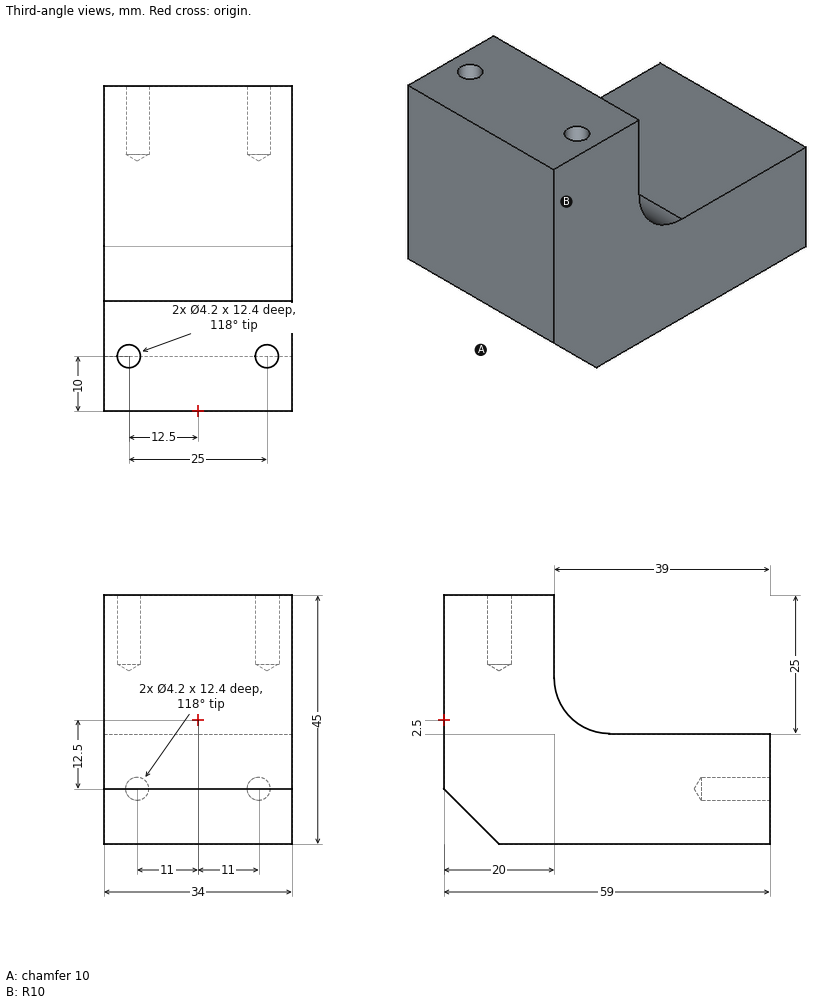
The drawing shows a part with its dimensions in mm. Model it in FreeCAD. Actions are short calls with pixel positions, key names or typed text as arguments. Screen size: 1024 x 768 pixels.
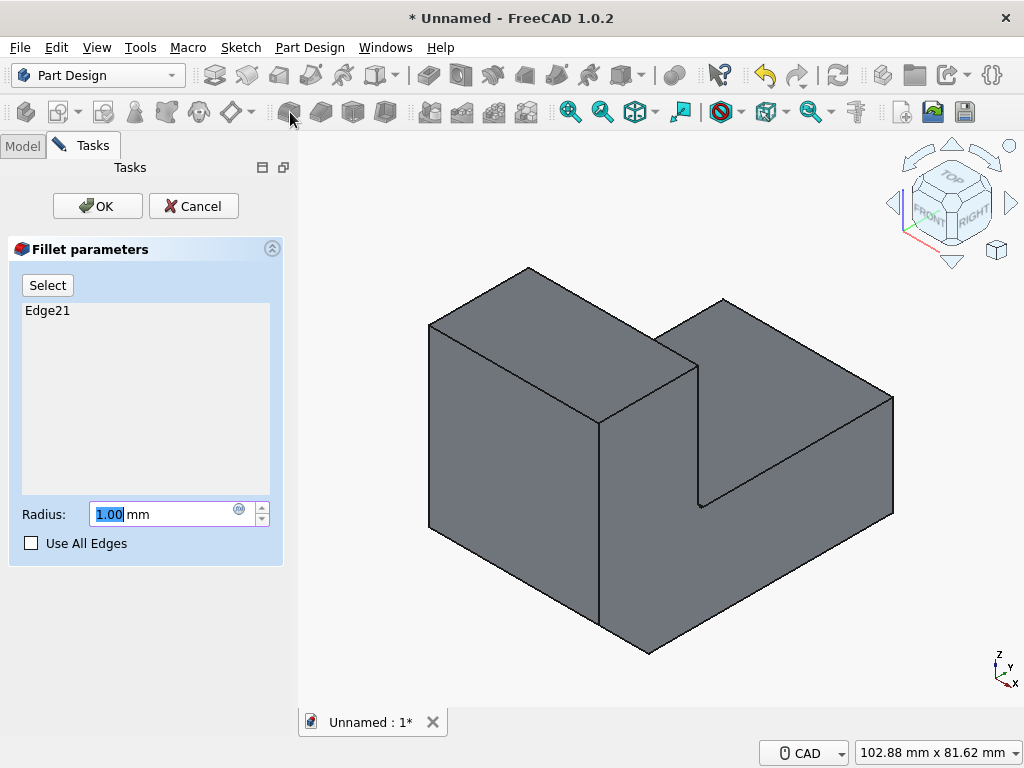
text(10)
key(Tab)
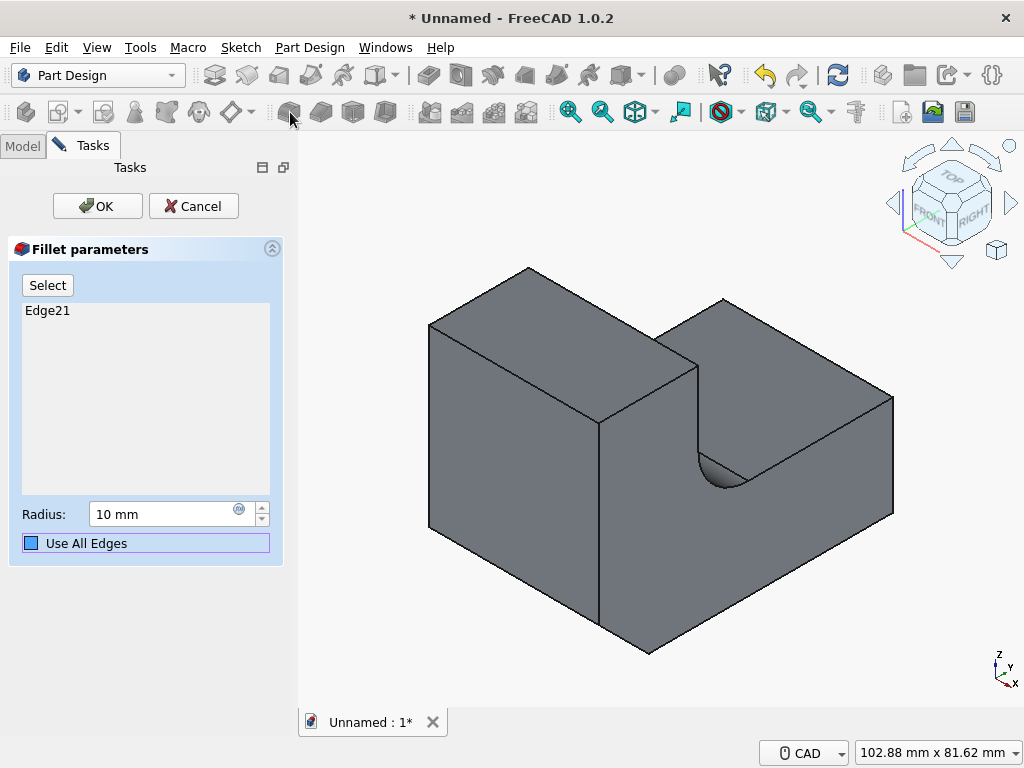
click(98, 206)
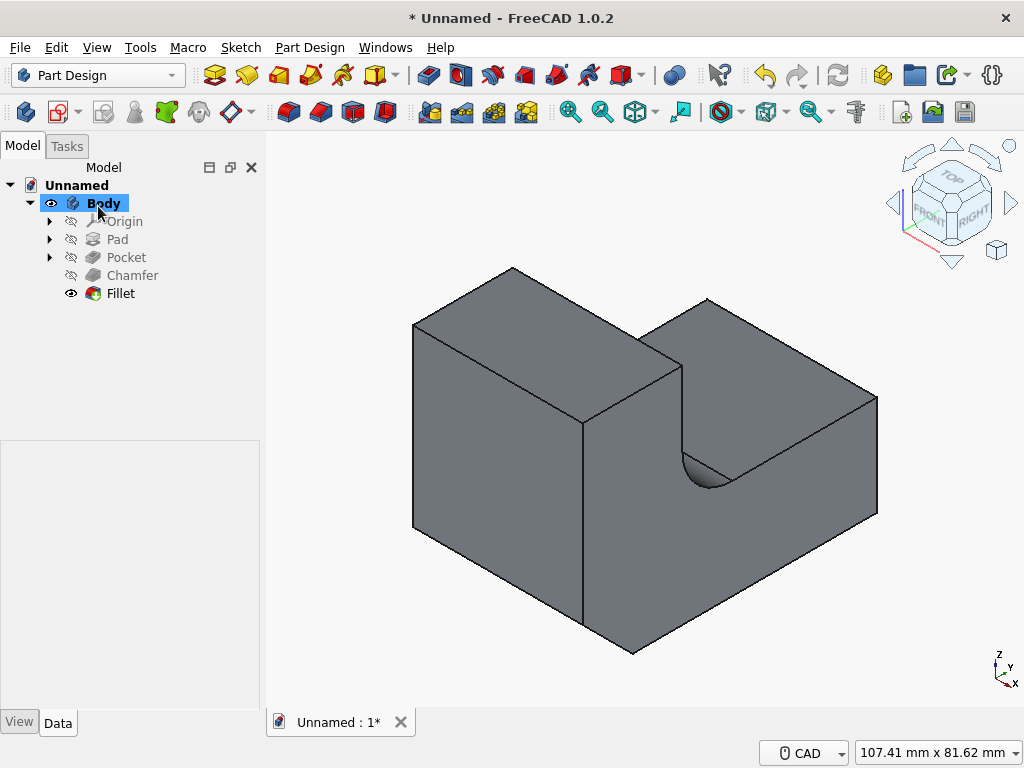
key(4)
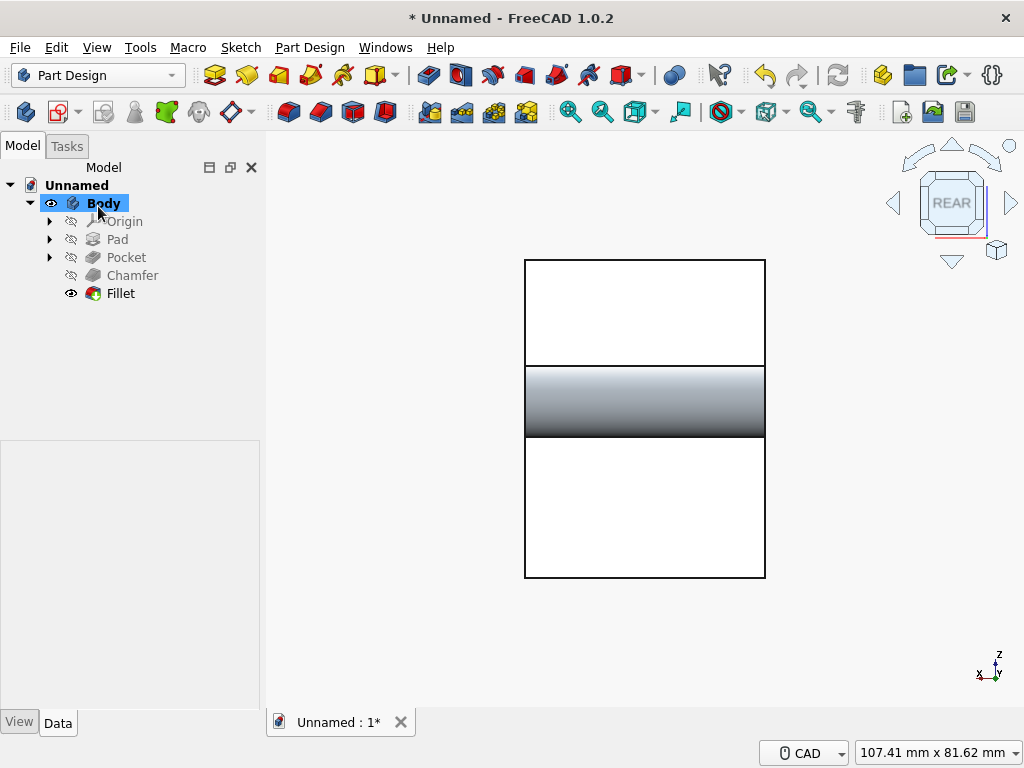
click(645, 506)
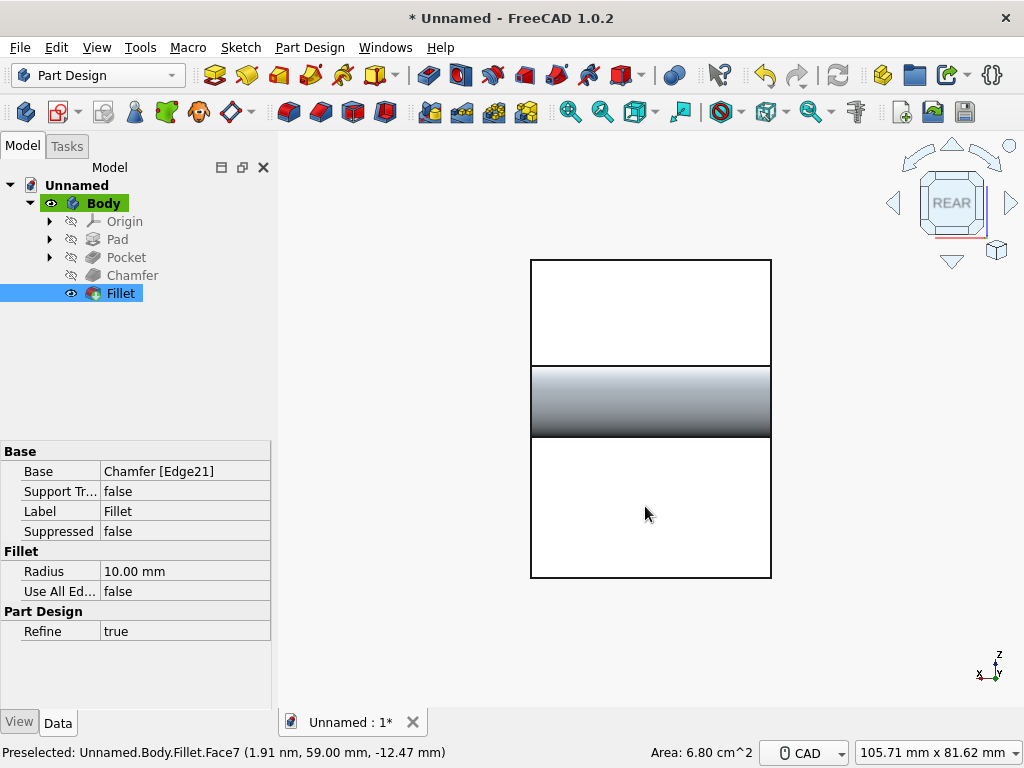
click(58, 112)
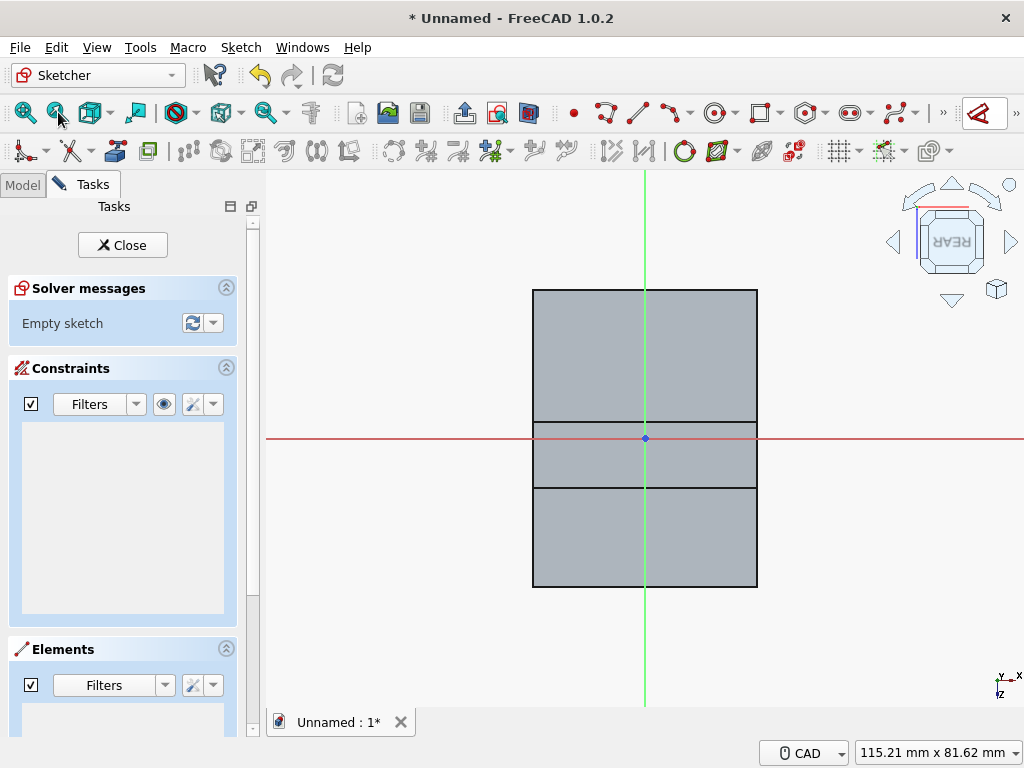
scroll(701, 351, up, 4)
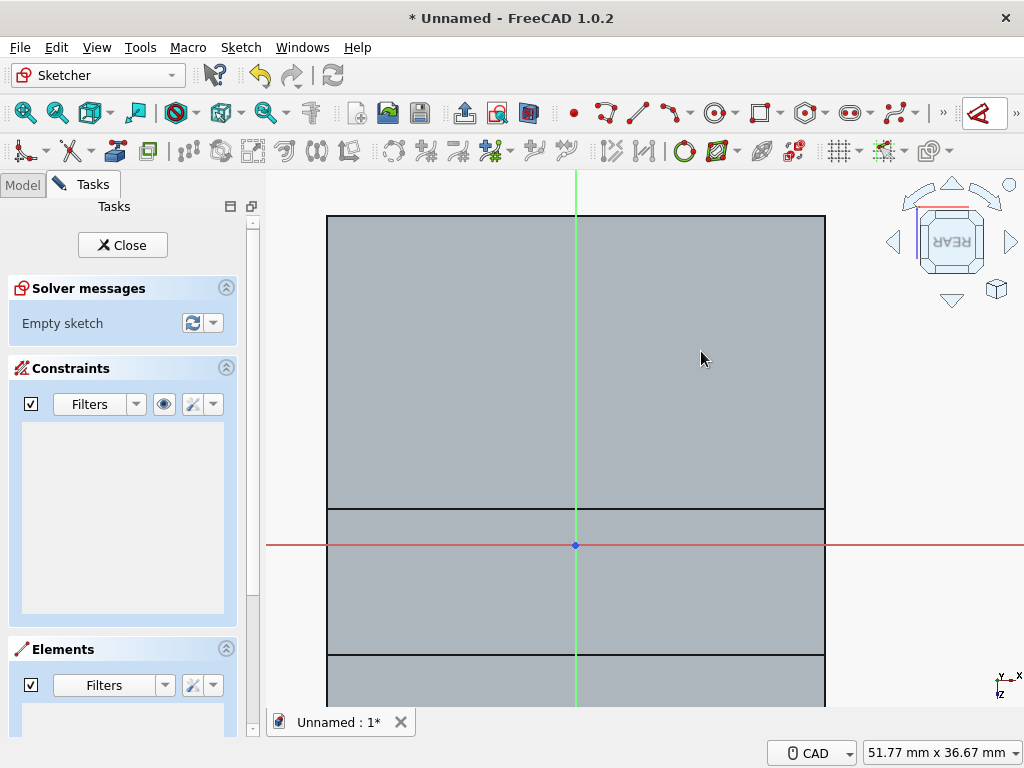
click(716, 114)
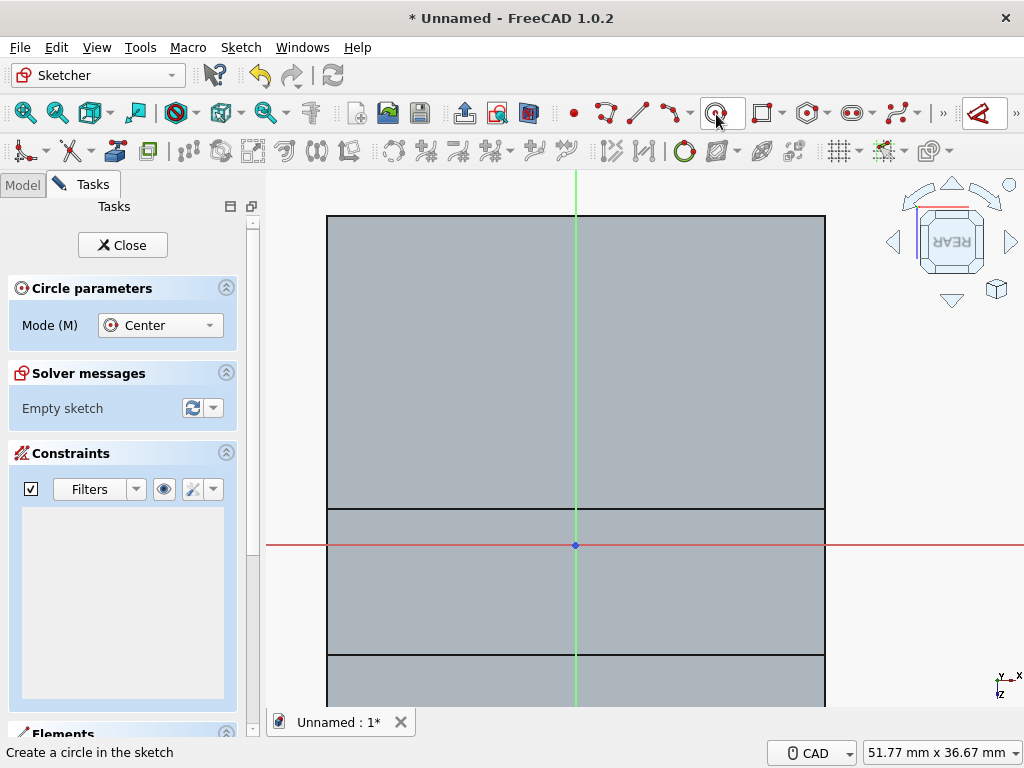
click(415, 362)
move(436, 341)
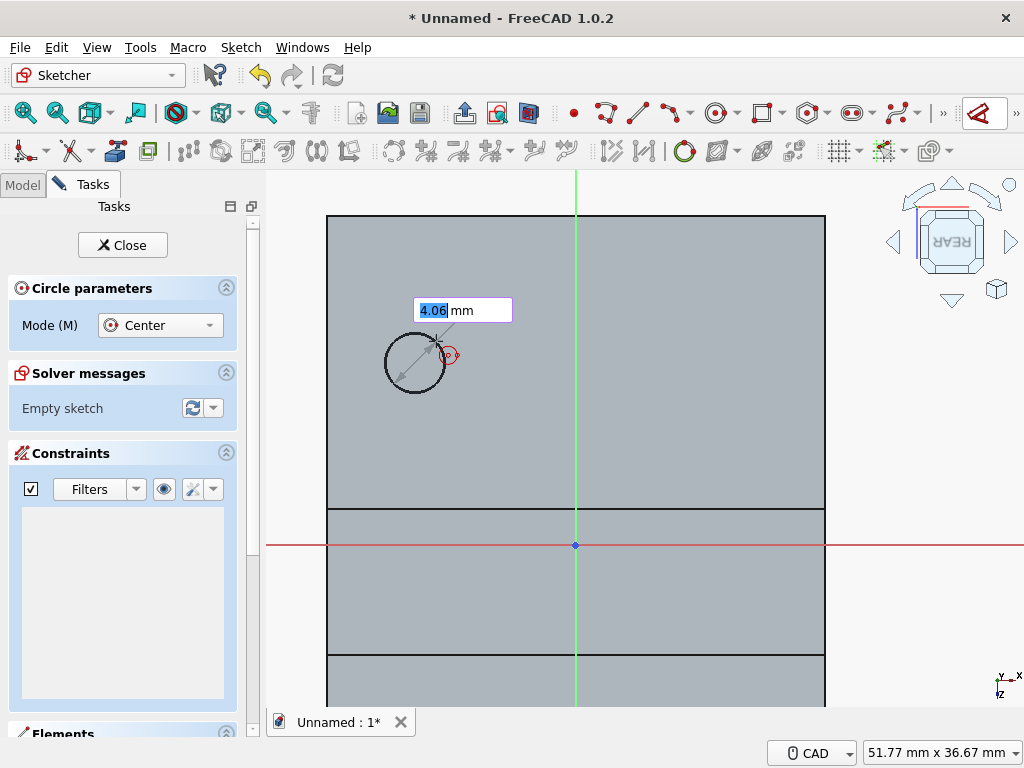
text(4.2)
key(Return)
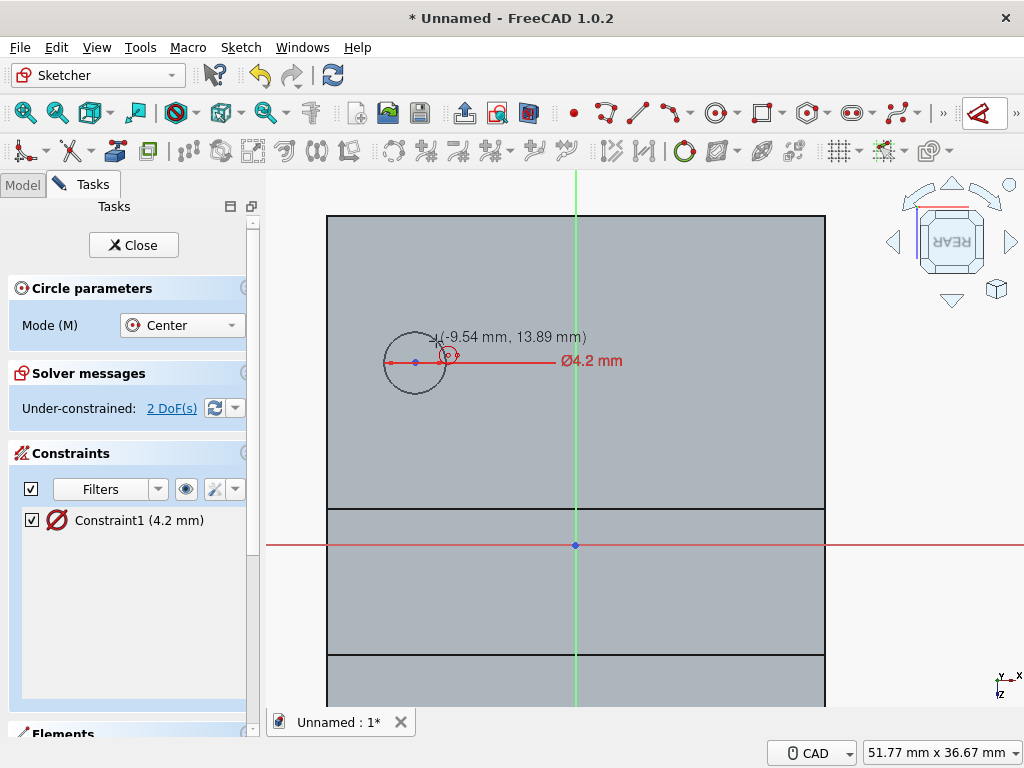
click(737, 362)
move(758, 341)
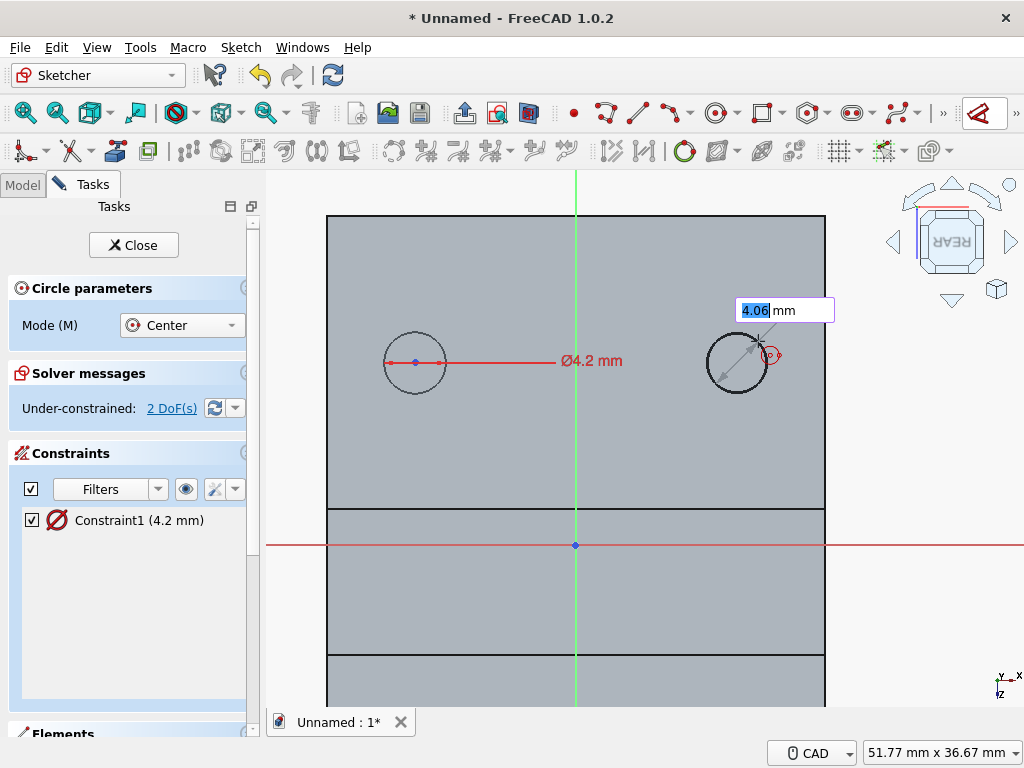
text(4.2)
key(Return)
key(Escape)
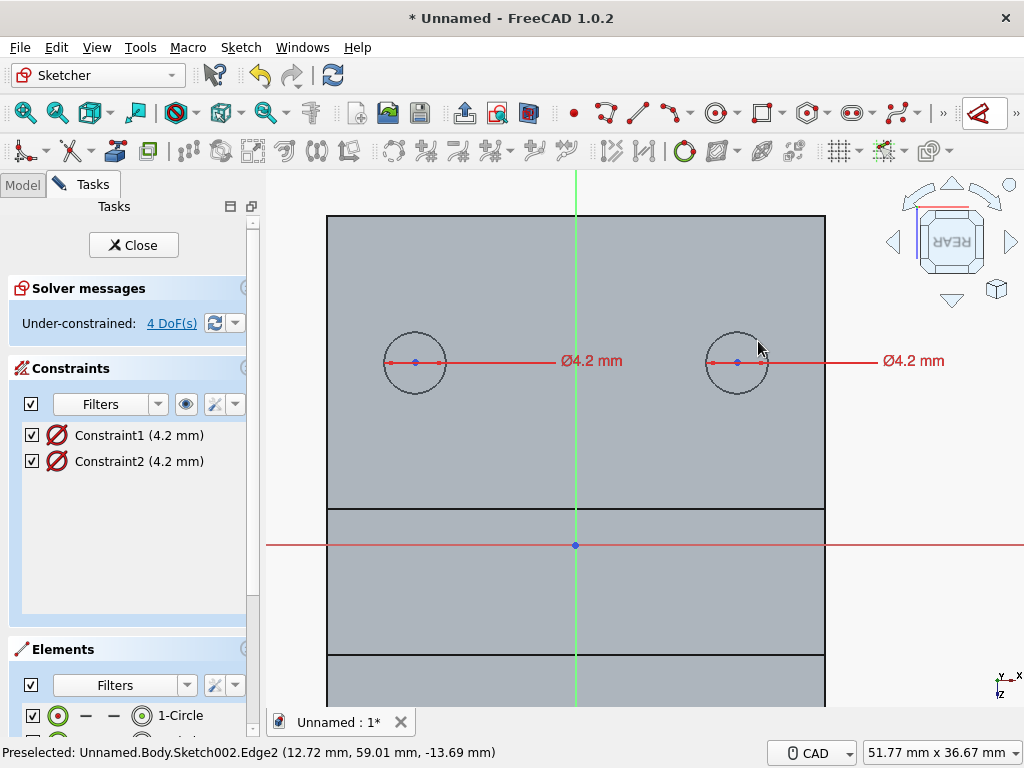
click(415, 363)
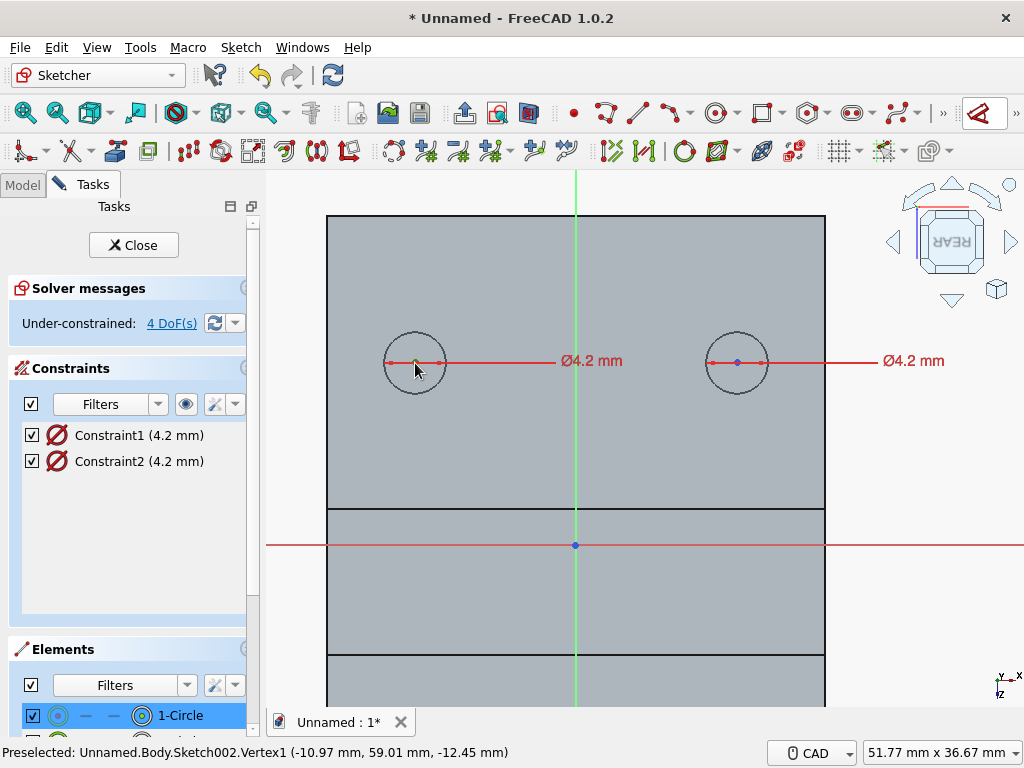
click(737, 363)